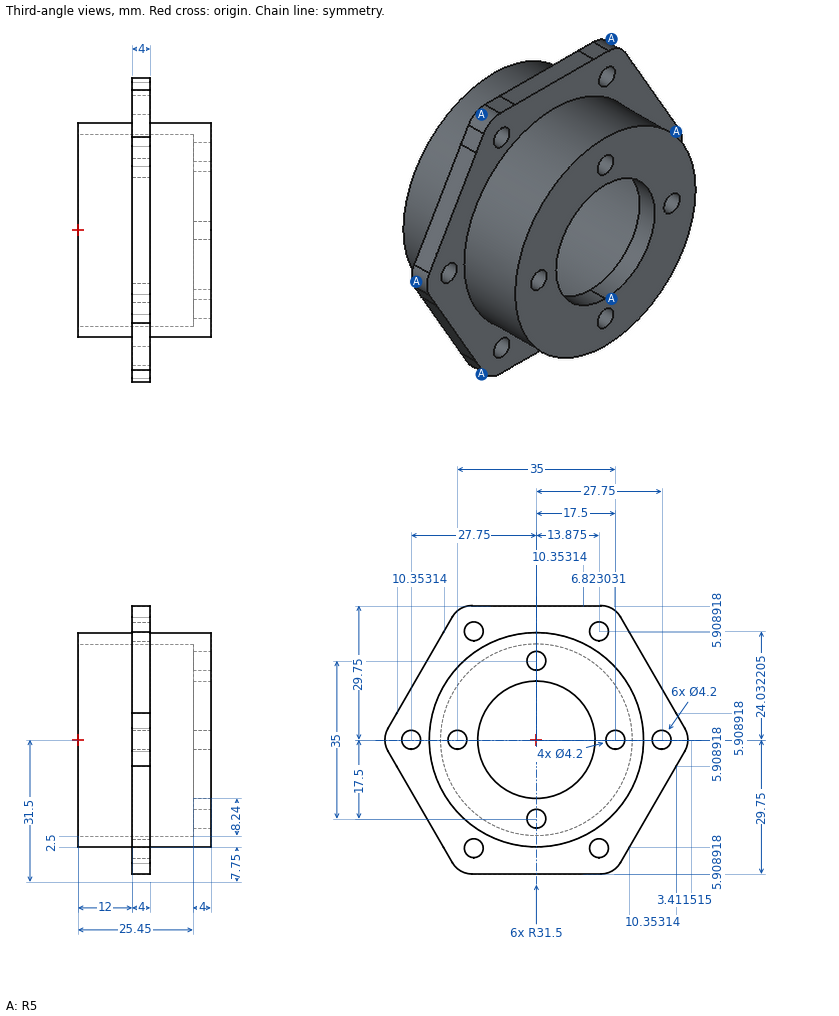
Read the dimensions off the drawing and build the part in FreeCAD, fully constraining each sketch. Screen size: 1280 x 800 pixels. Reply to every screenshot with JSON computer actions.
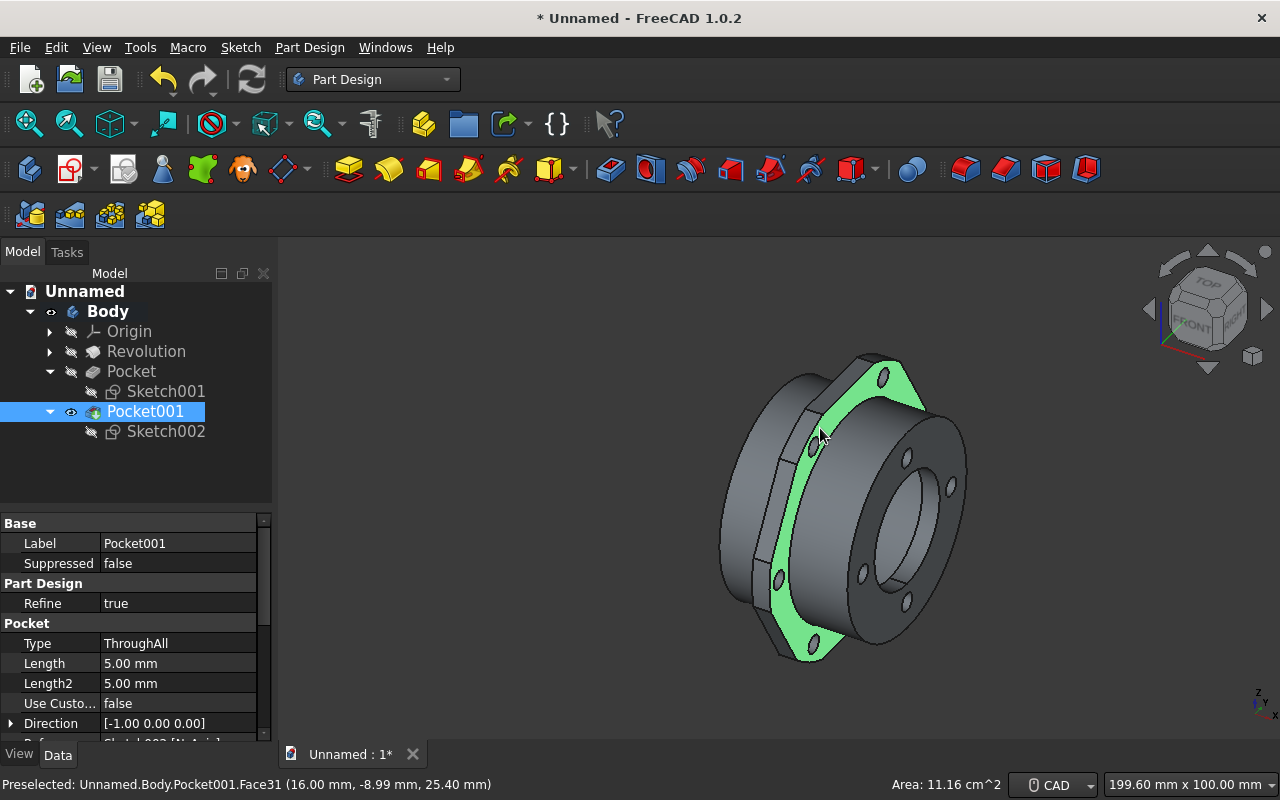
{"action": "left_click", "coordinate": [70, 170]}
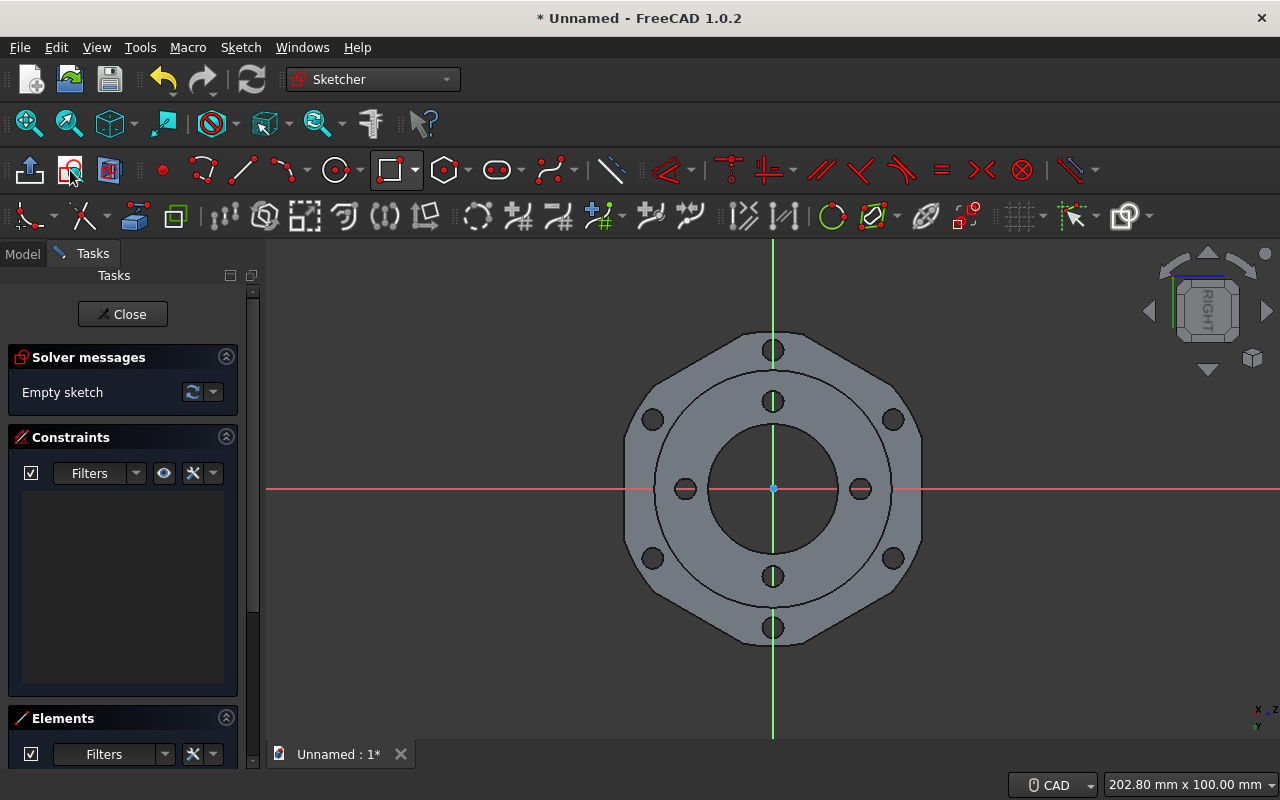
{"action": "left_click", "coordinate": [204, 170]}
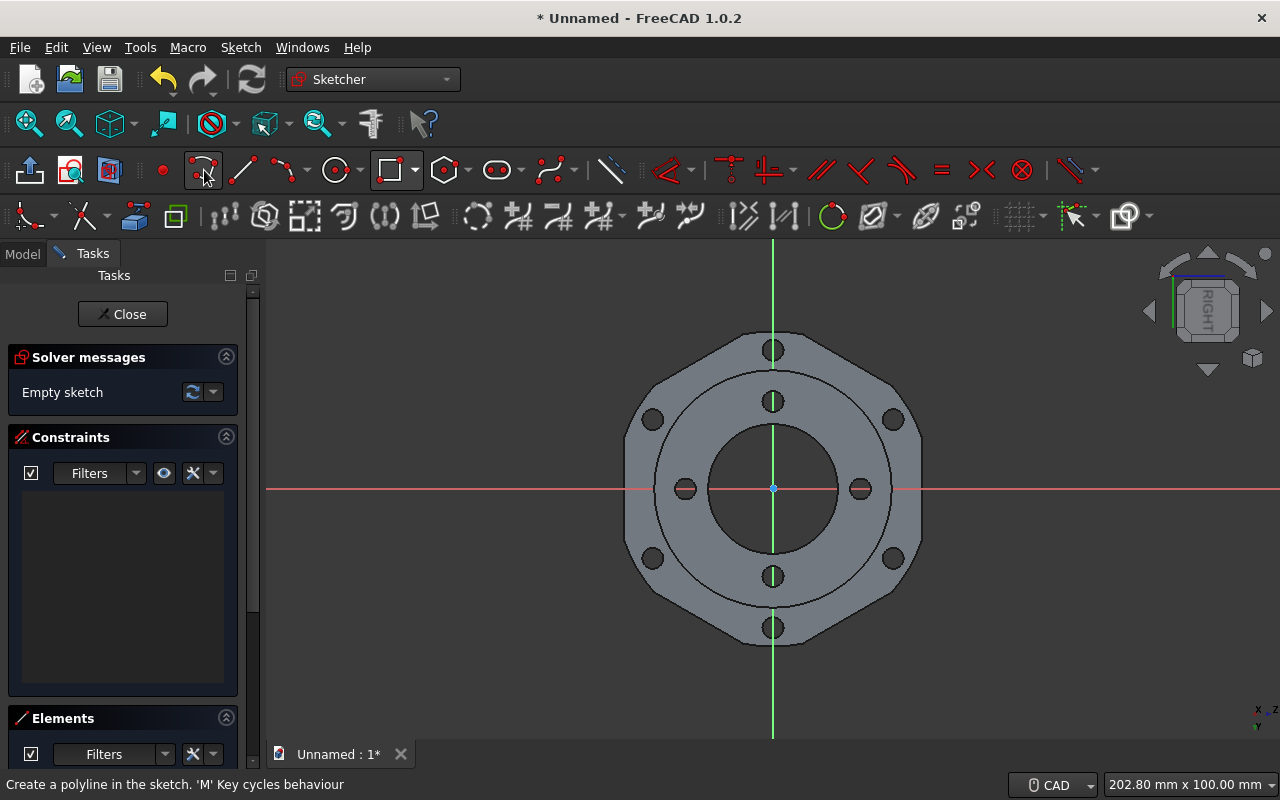
{"action": "left_click", "coordinate": [892, 592]}
{"action": "left_click", "coordinate": [922, 575]}
{"action": "left_click", "coordinate": [922, 541]}
{"action": "right_click", "coordinate": [922, 541]}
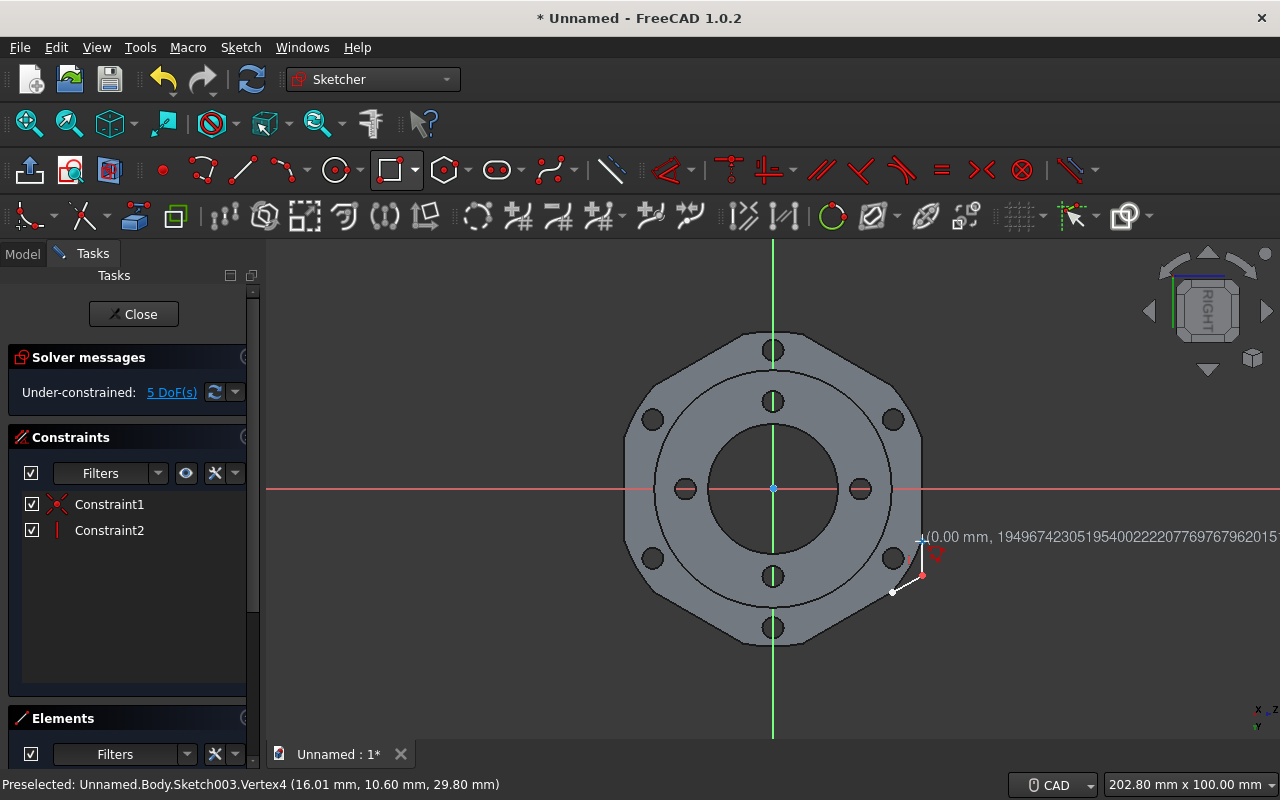
{"action": "key", "text": "g 3 a"}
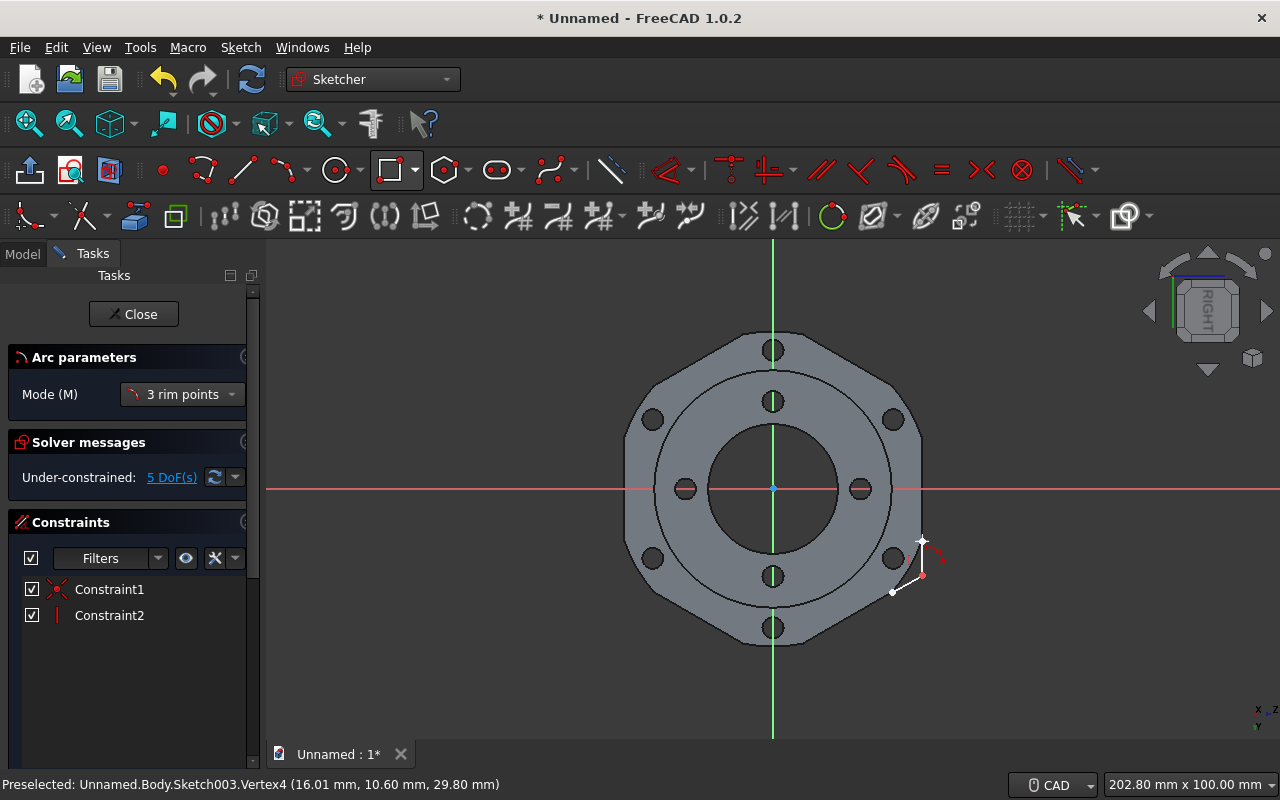
{"action": "left_click", "coordinate": [922, 542]}
{"action": "left_click", "coordinate": [892, 593]}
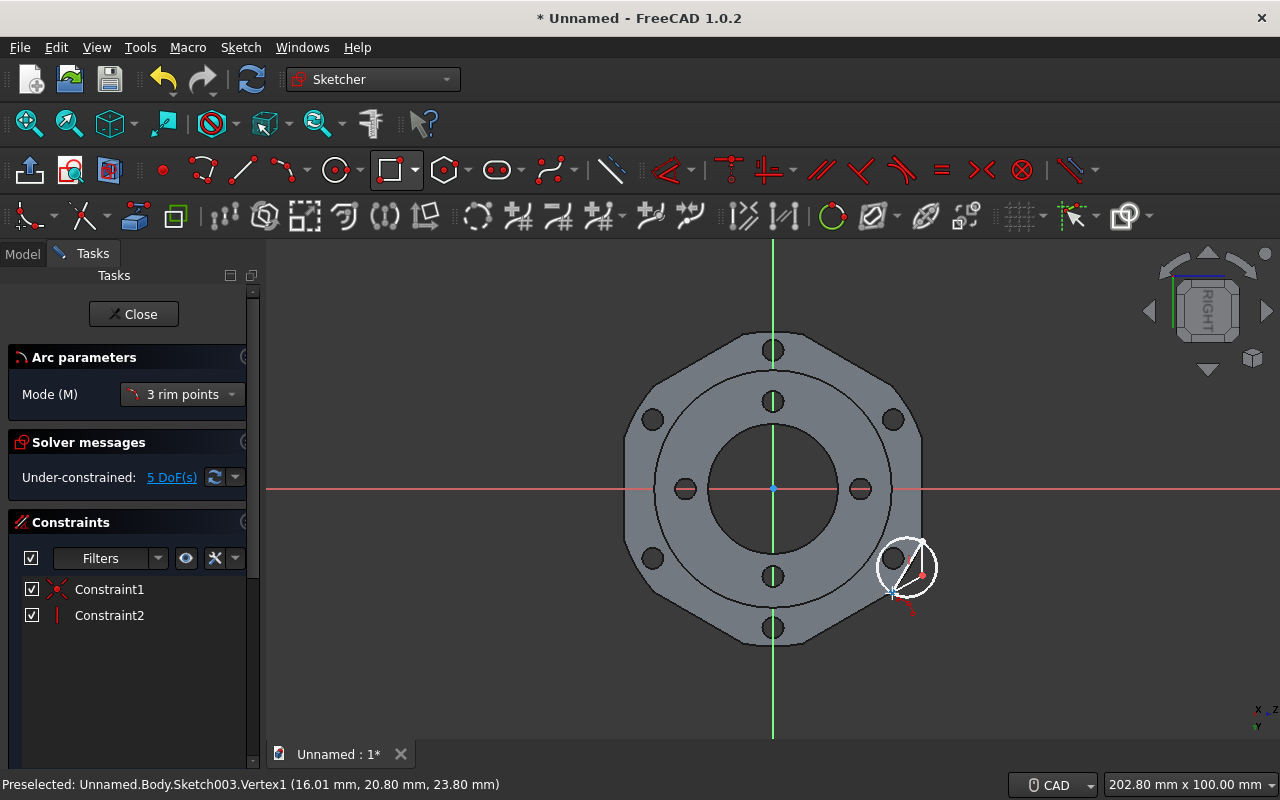
{"action": "scroll", "coordinate": [909, 568], "scroll_direction": "up", "scroll_amount": 9}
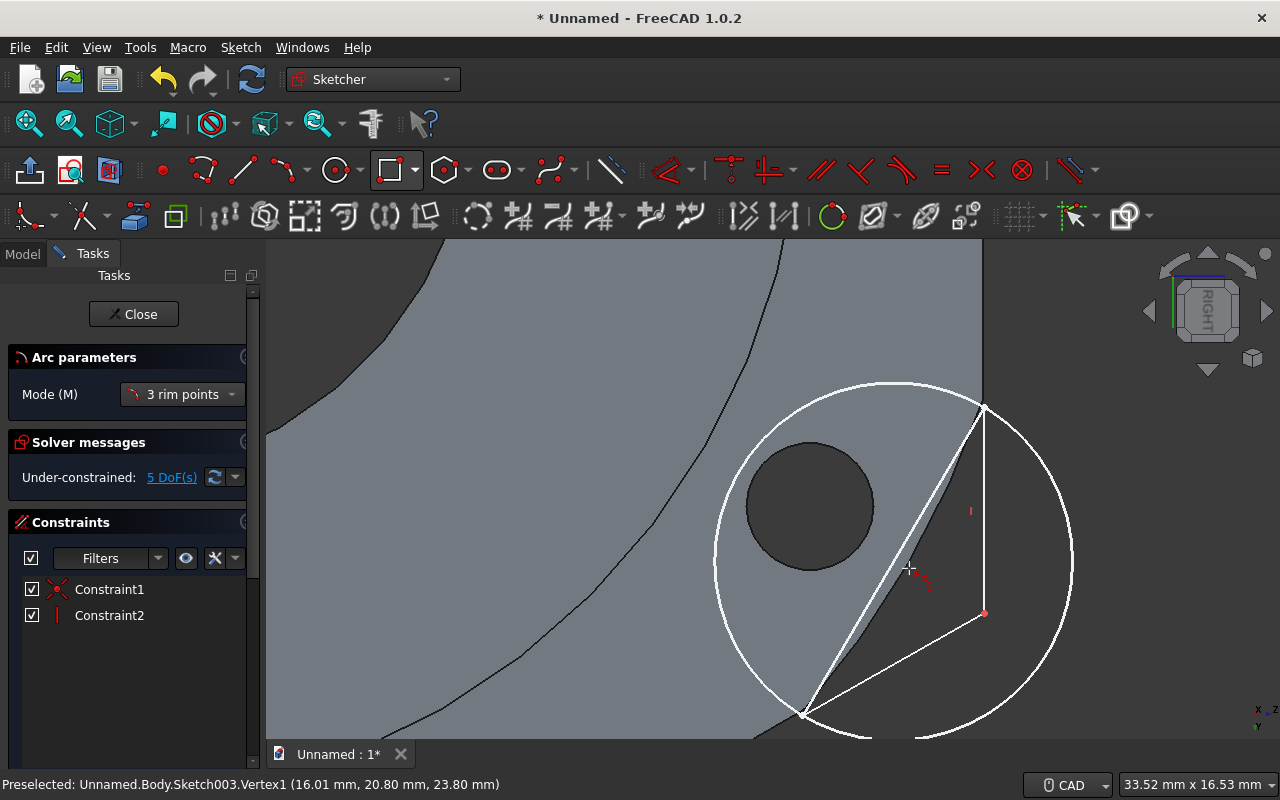
{"action": "left_click", "coordinate": [908, 563]}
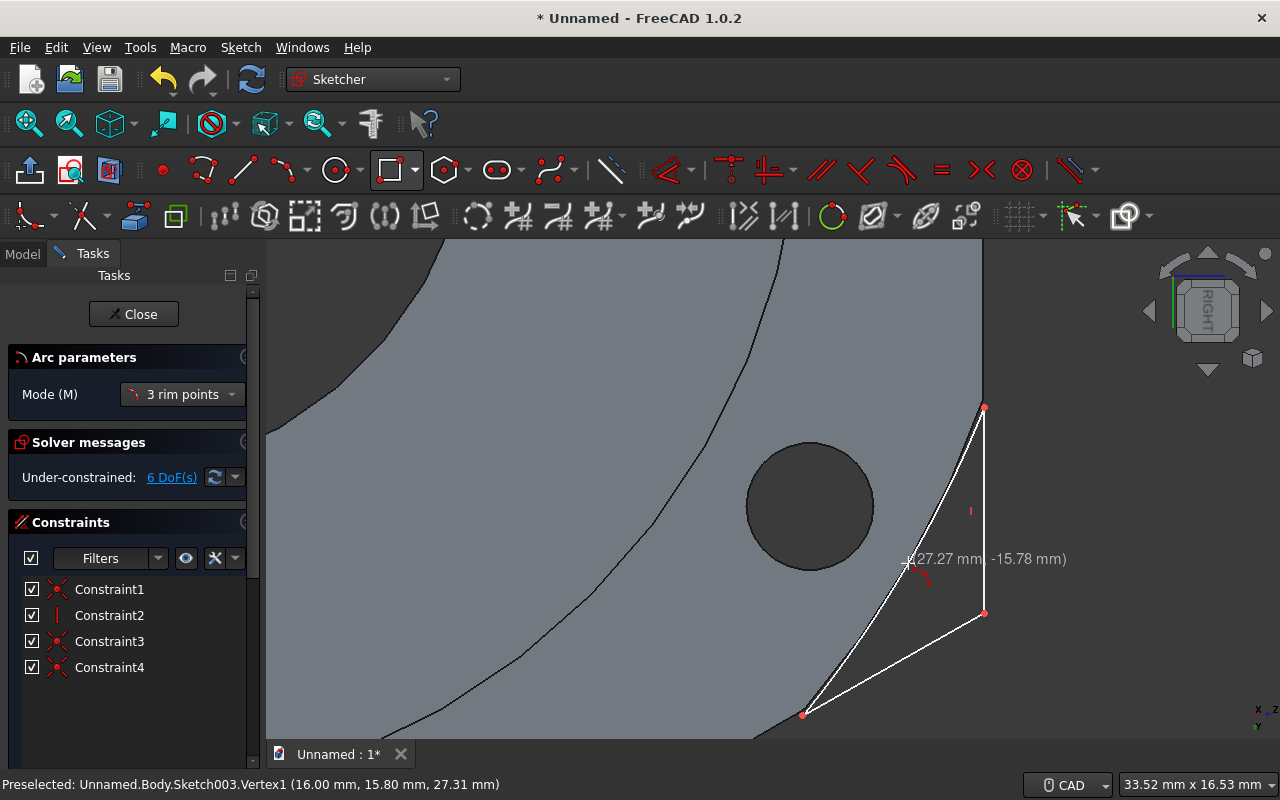
{"action": "key", "text": "g m"}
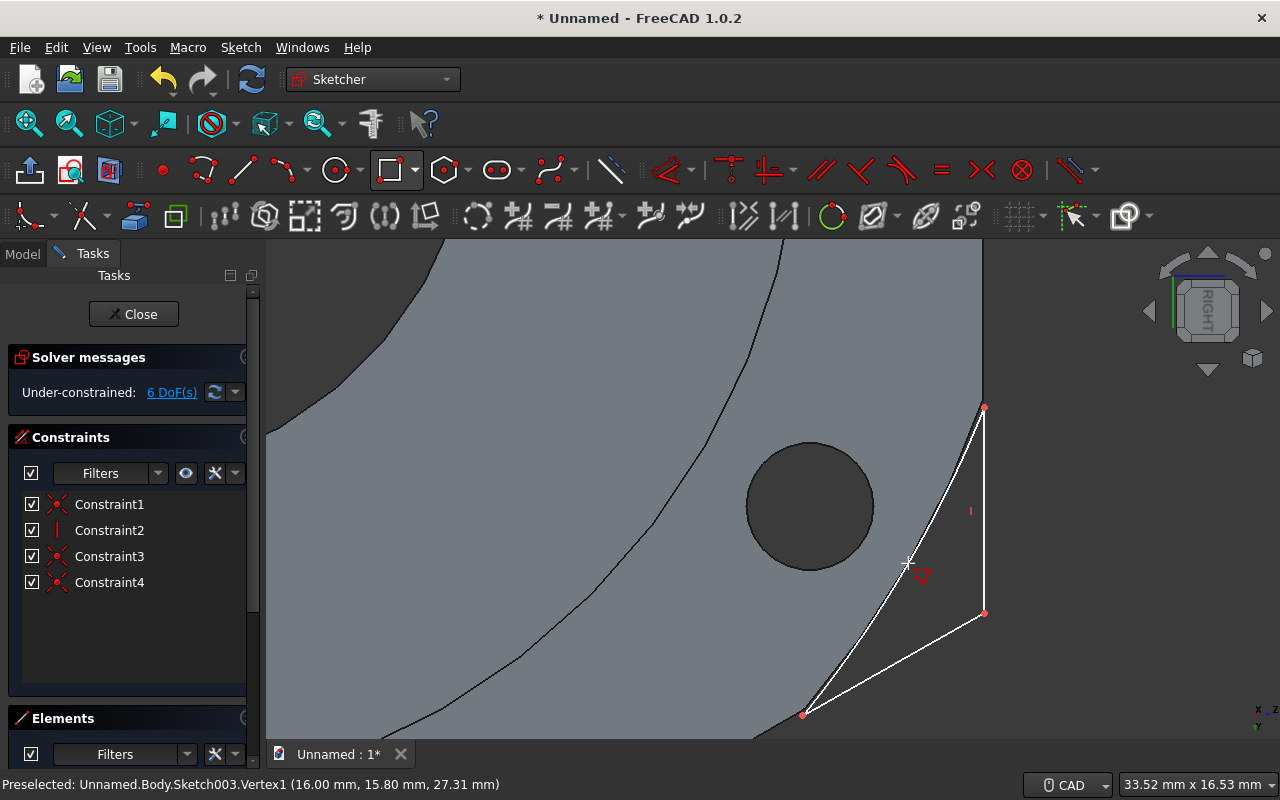
{"action": "scroll", "coordinate": [828, 569], "scroll_direction": "down", "scroll_amount": 9}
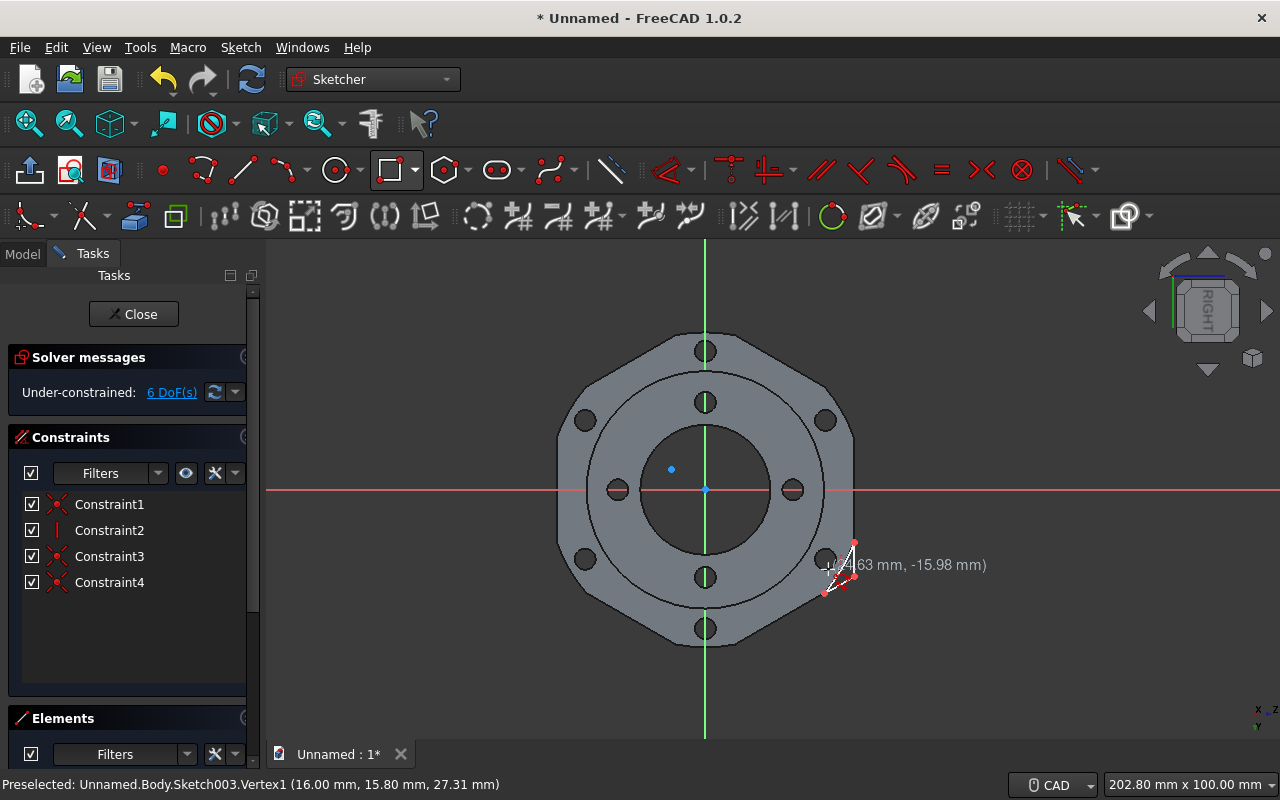
{"action": "left_click", "coordinate": [676, 645]}
{"action": "left_click", "coordinate": [705, 662]}
{"action": "left_click", "coordinate": [735, 645]}
{"action": "right_click", "coordinate": [735, 645]}